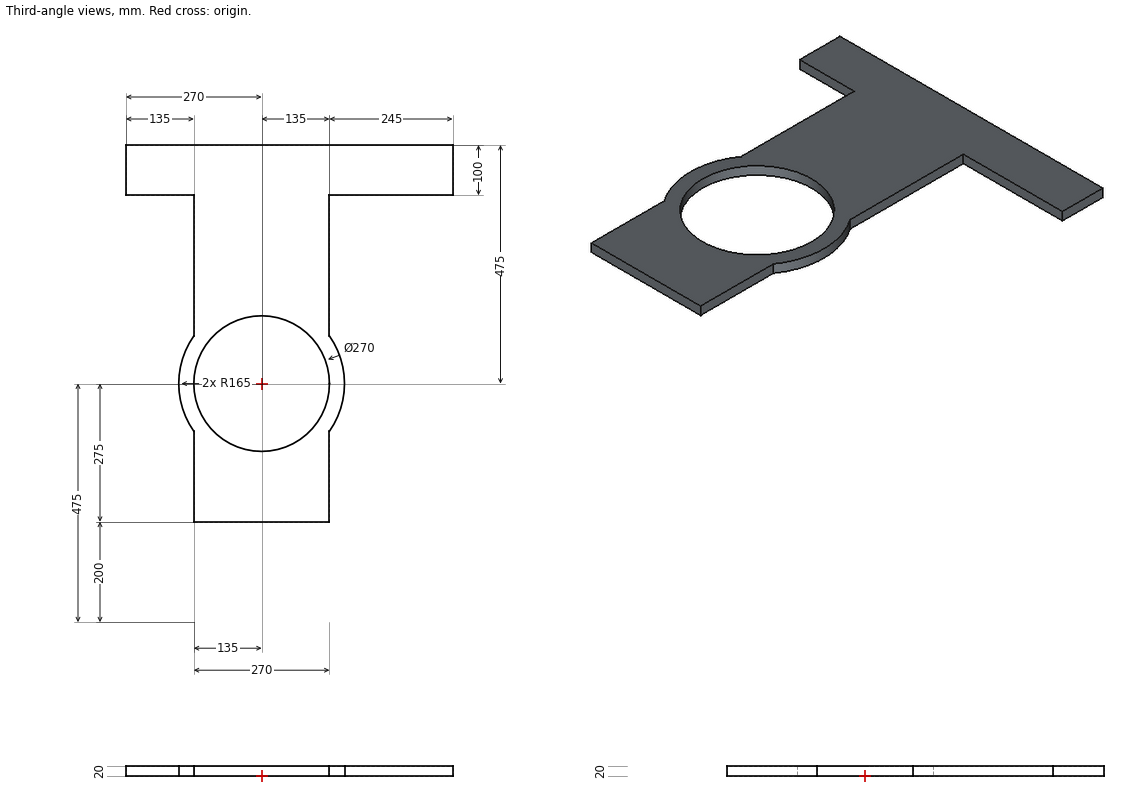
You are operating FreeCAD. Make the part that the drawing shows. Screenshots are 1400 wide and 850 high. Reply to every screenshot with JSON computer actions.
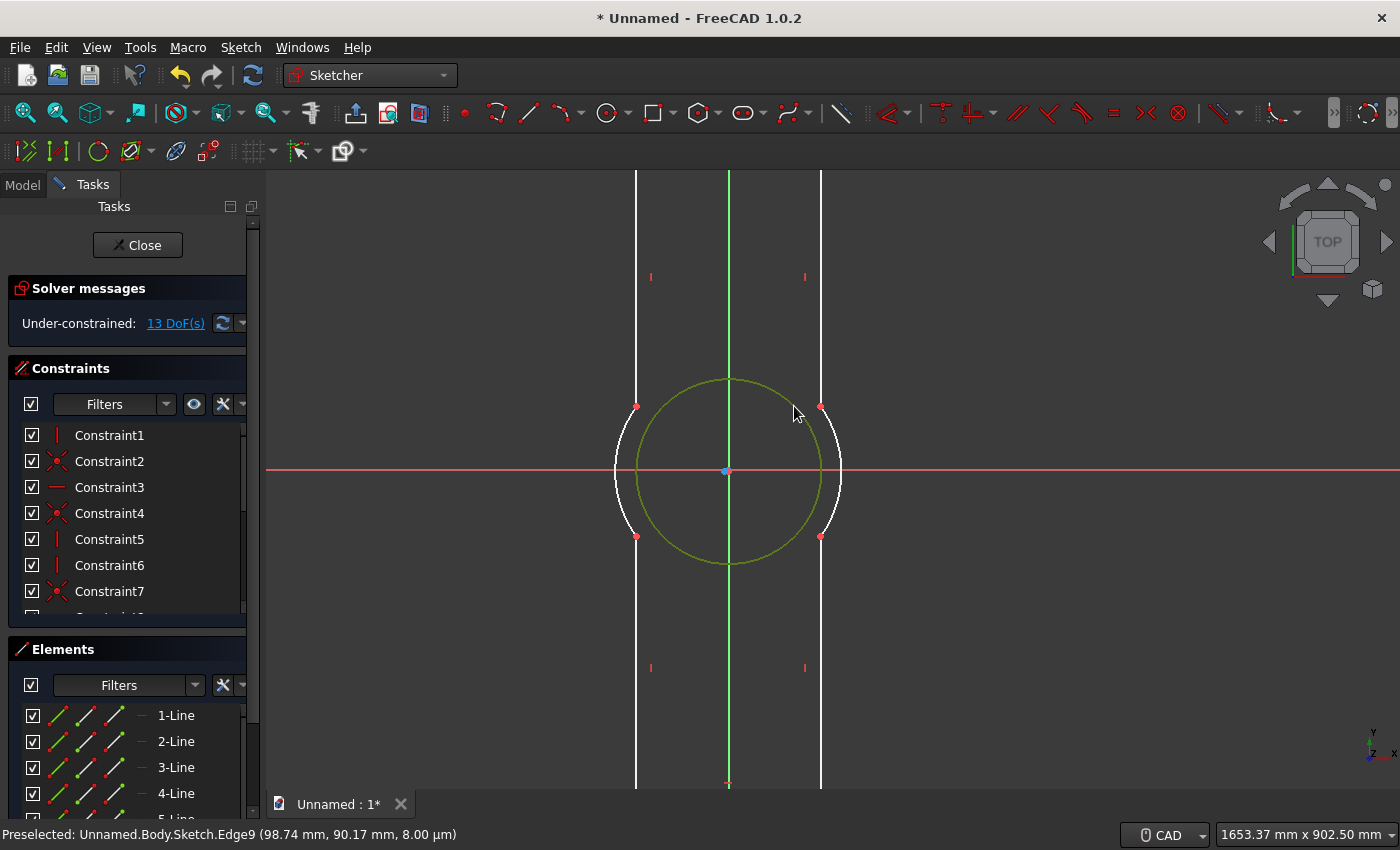
{"action": "left_click", "coordinate": [619, 444]}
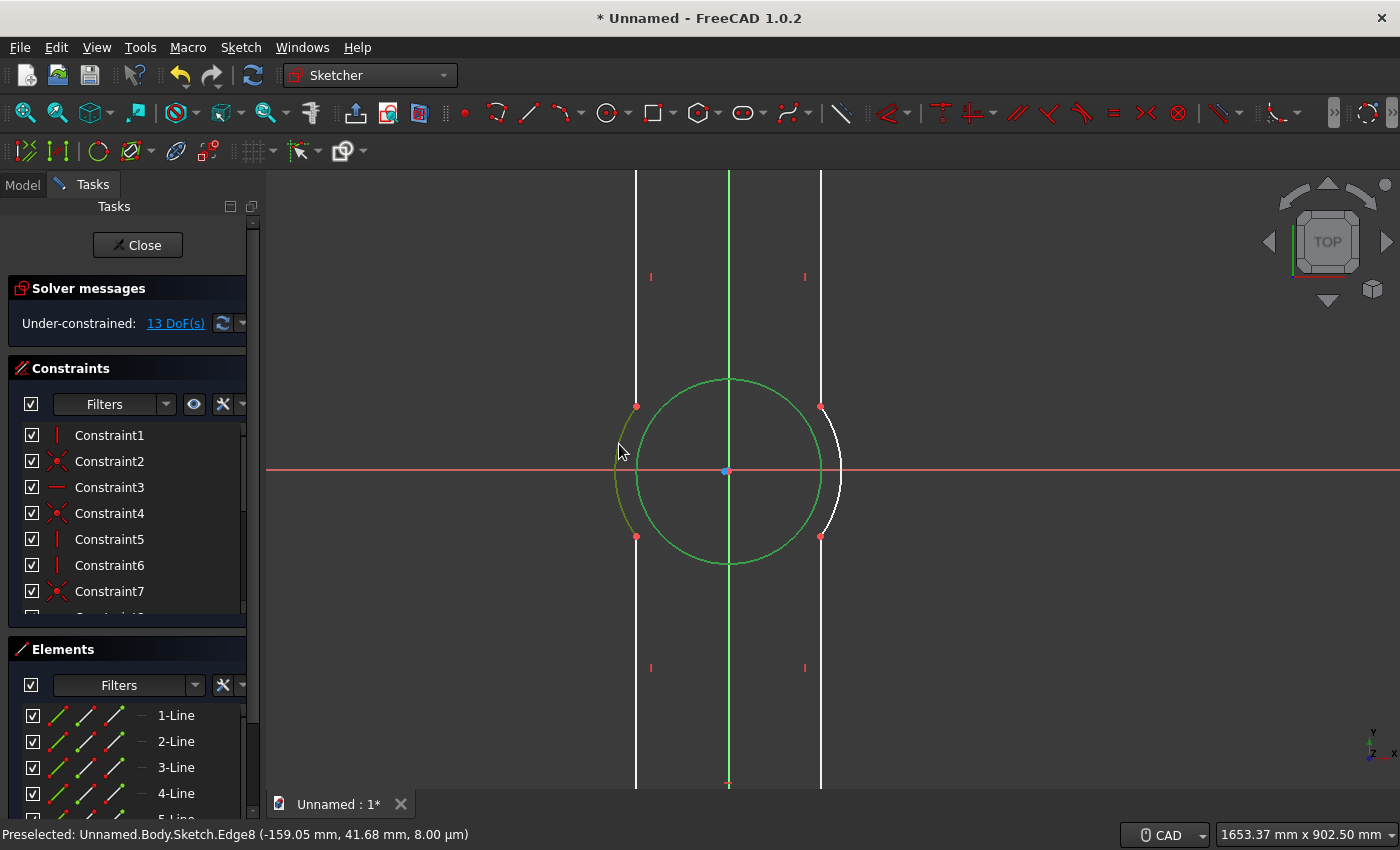
{"action": "key", "text": "c"}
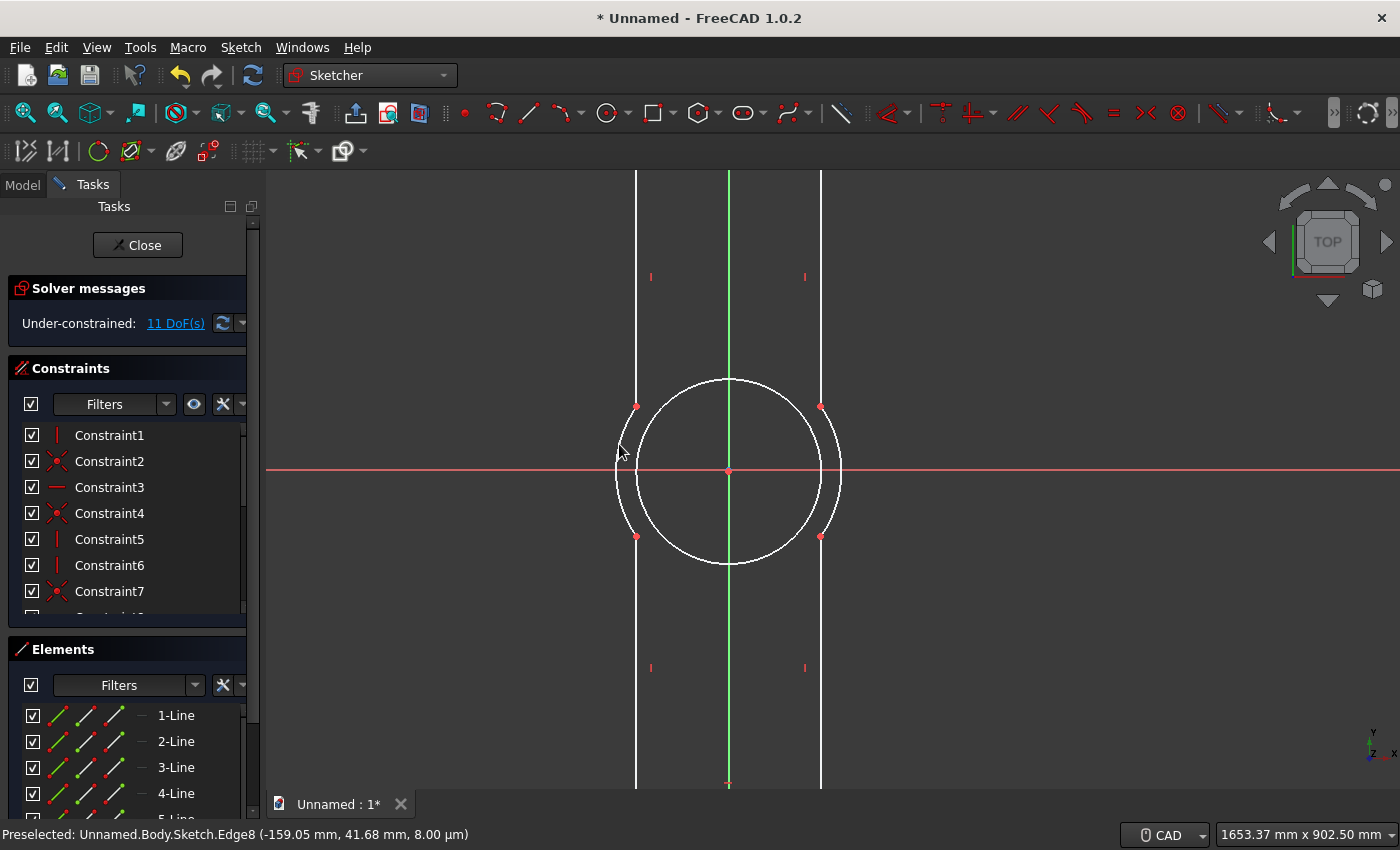
{"action": "left_click_drag", "start_coordinate": [719, 460], "coordinate": [739, 482]}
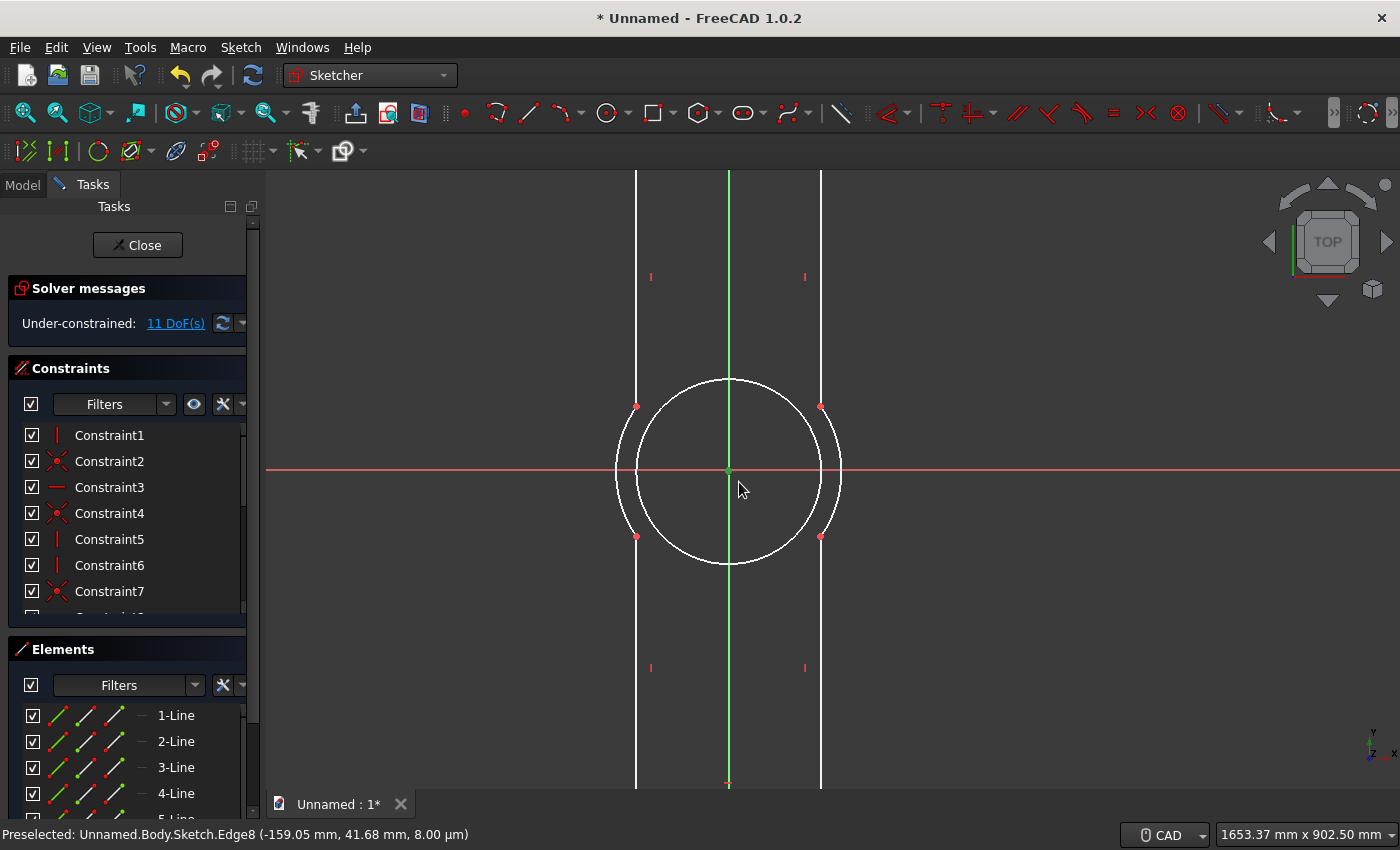
{"action": "left_click", "coordinate": [942, 114]}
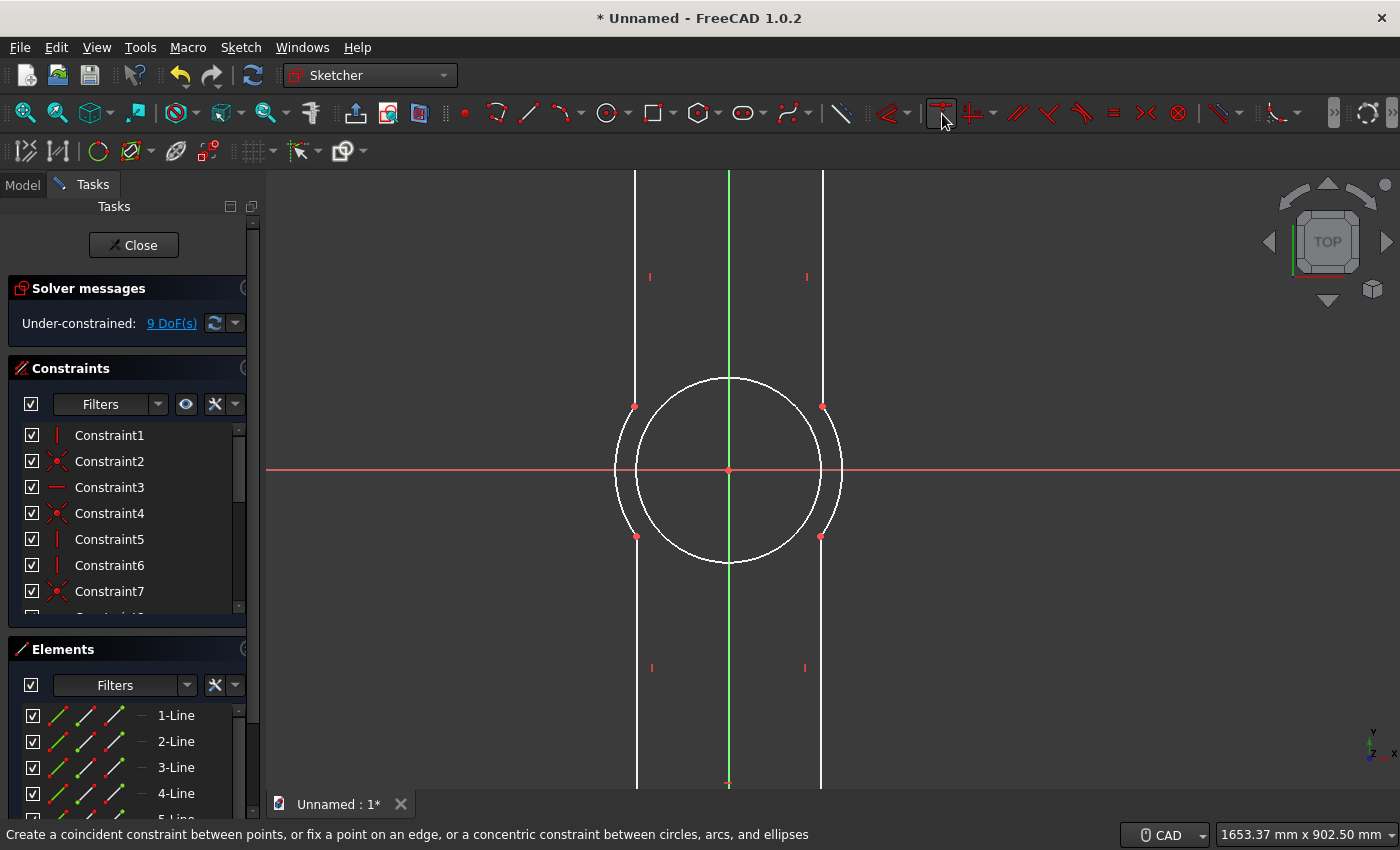
{"action": "left_click", "coordinate": [838, 499]}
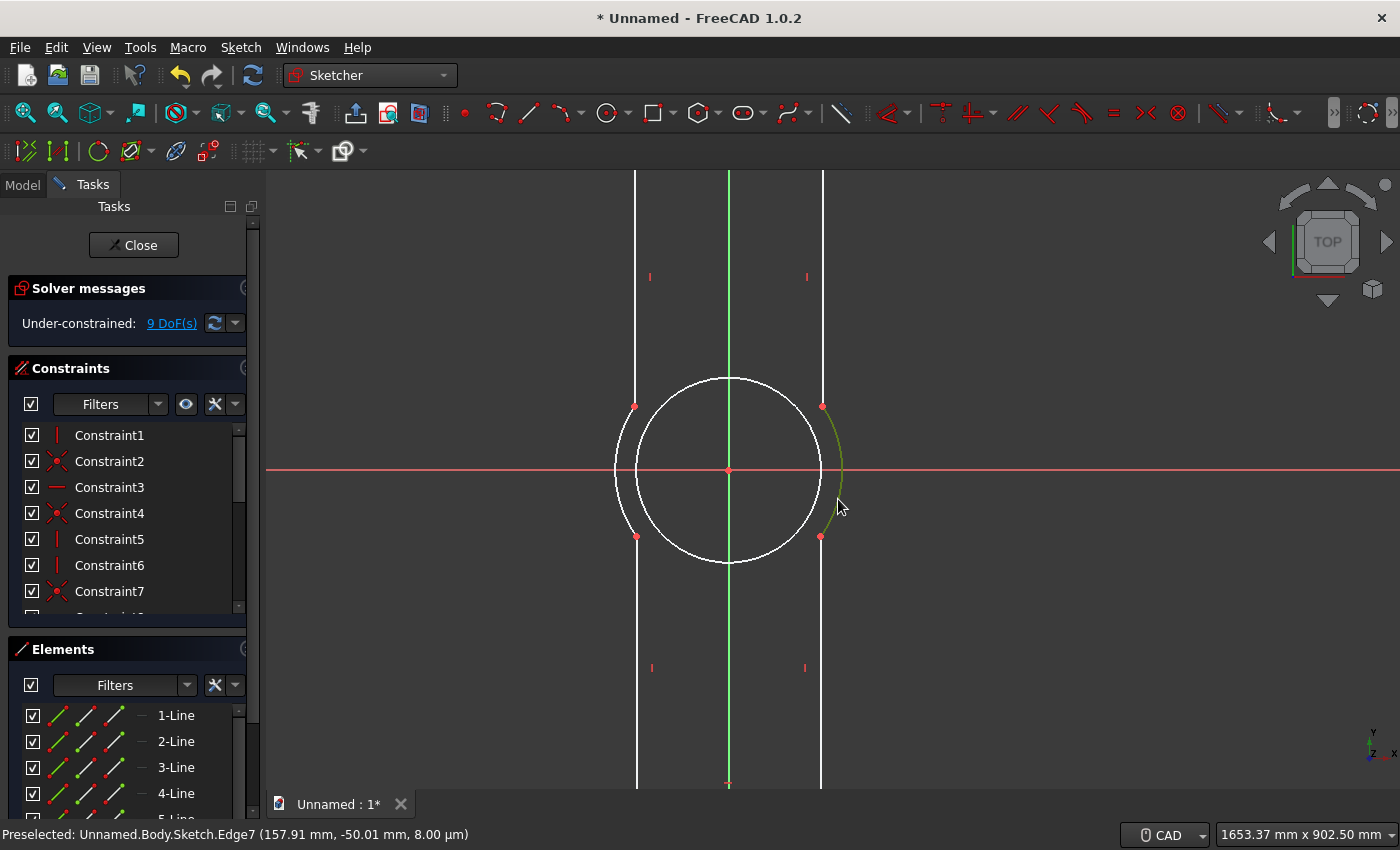
{"action": "left_click", "coordinate": [618, 445]}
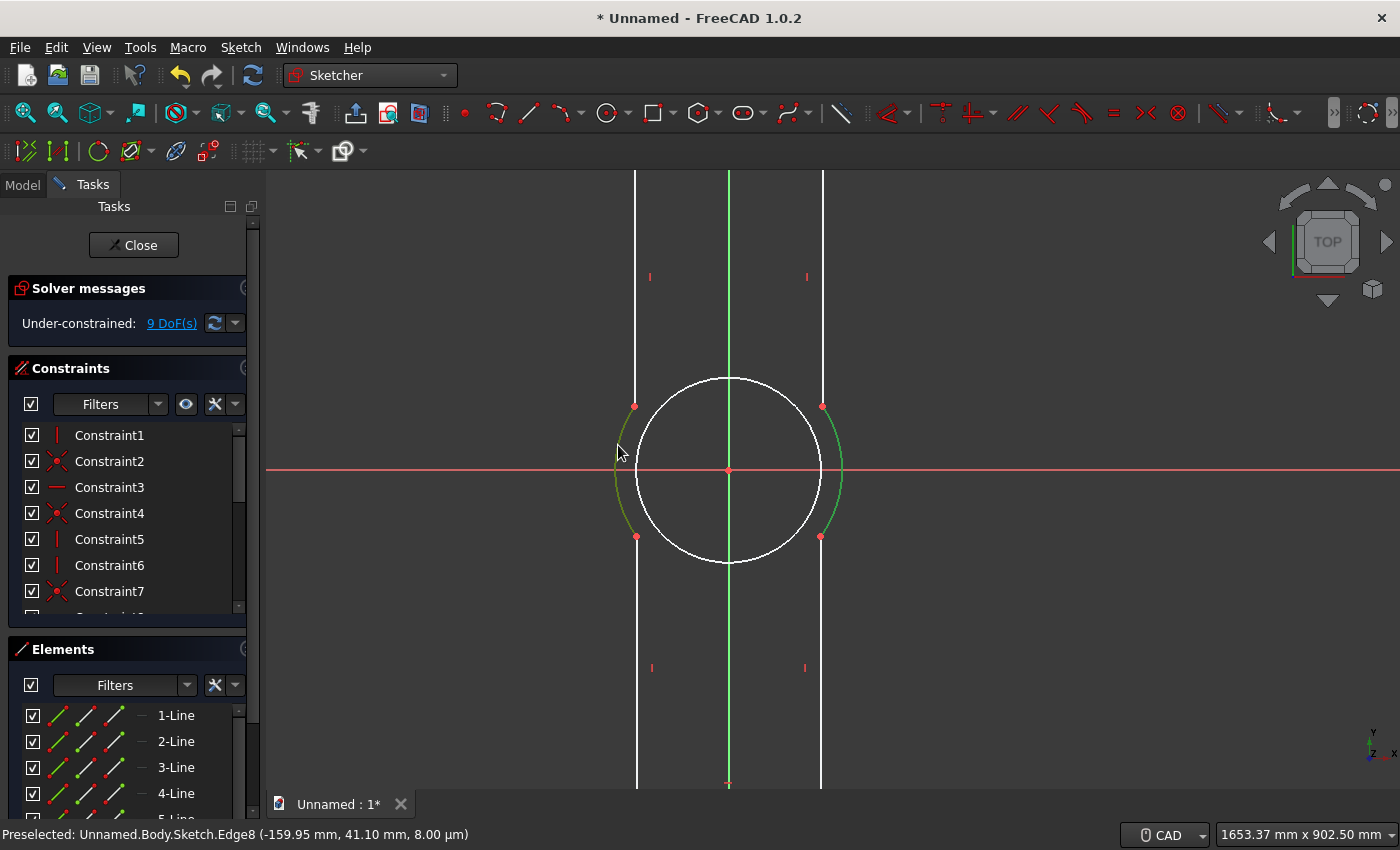
{"action": "key", "text": "e"}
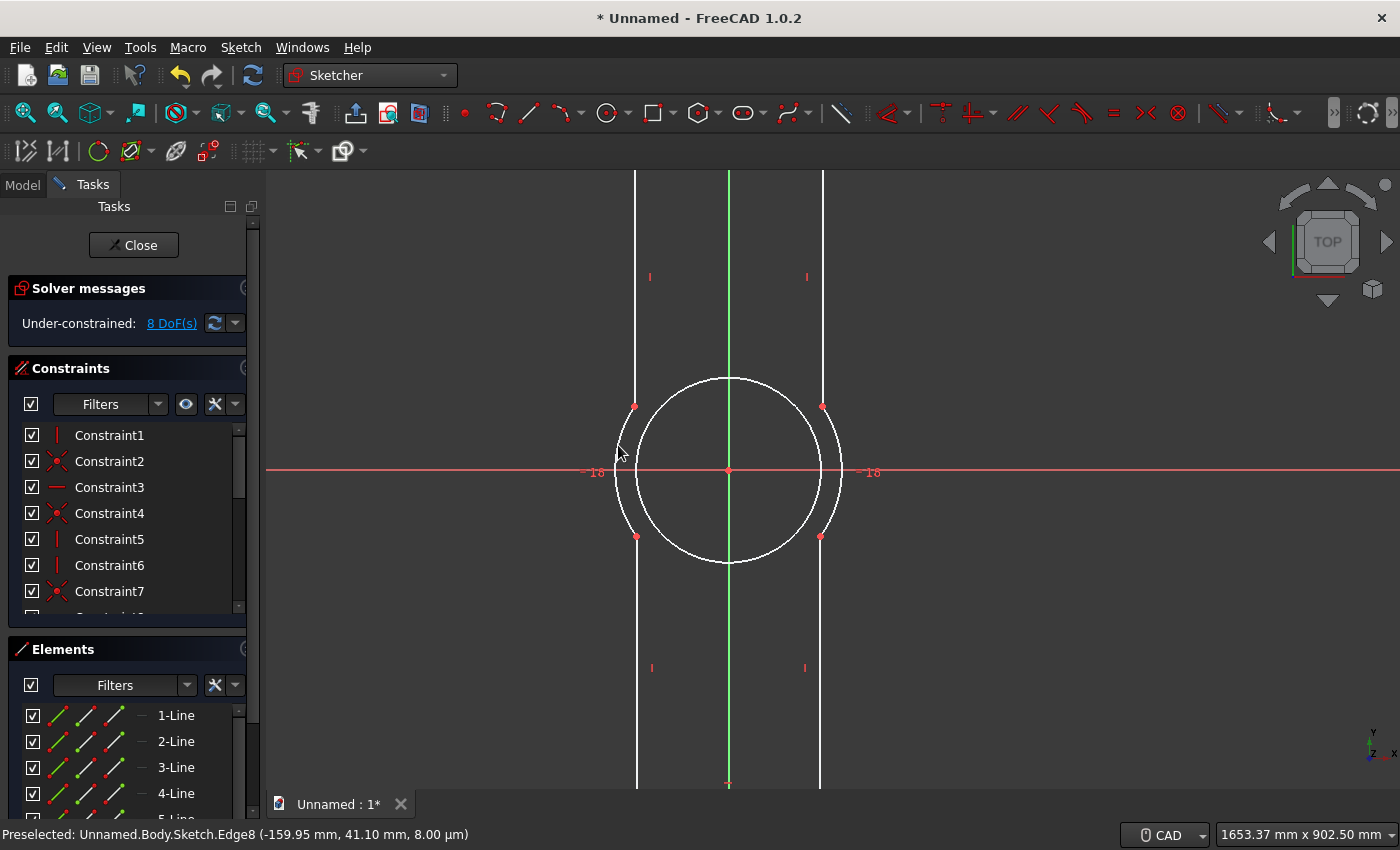
{"action": "key", "text": "d"}